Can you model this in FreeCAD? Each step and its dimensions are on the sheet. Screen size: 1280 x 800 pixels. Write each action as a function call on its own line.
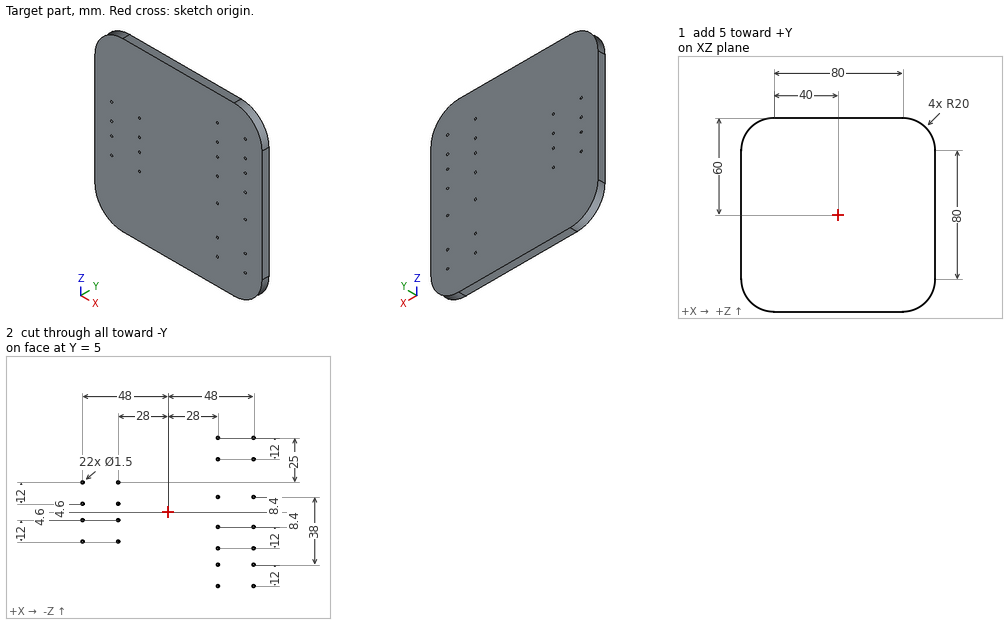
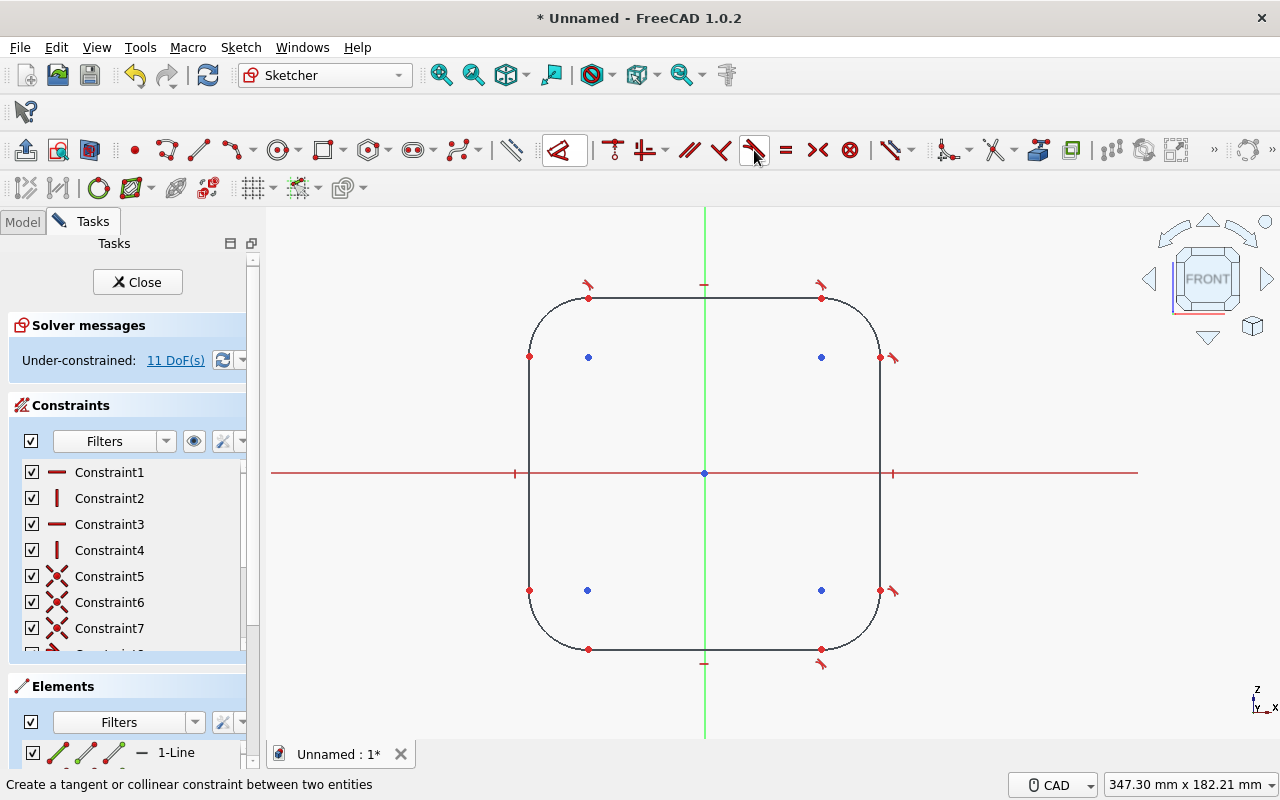
click(751, 650)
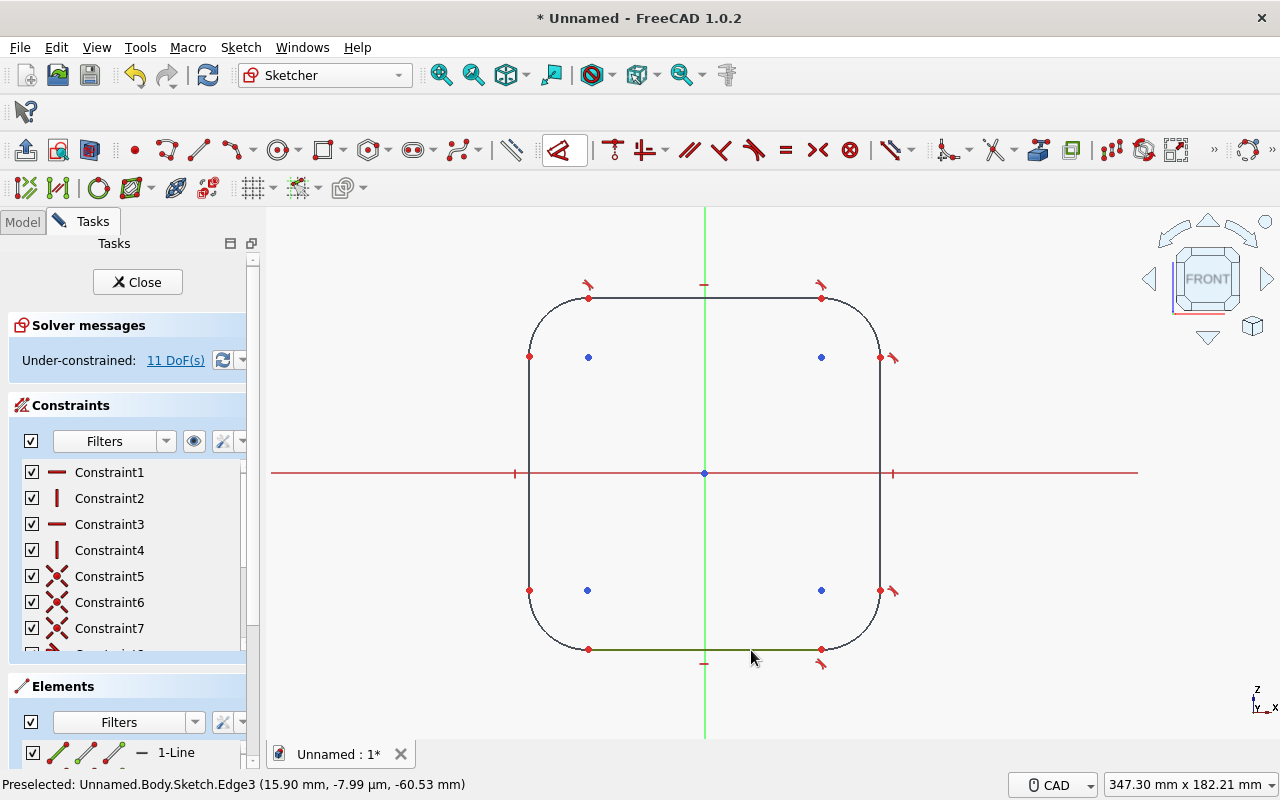
click(535, 618)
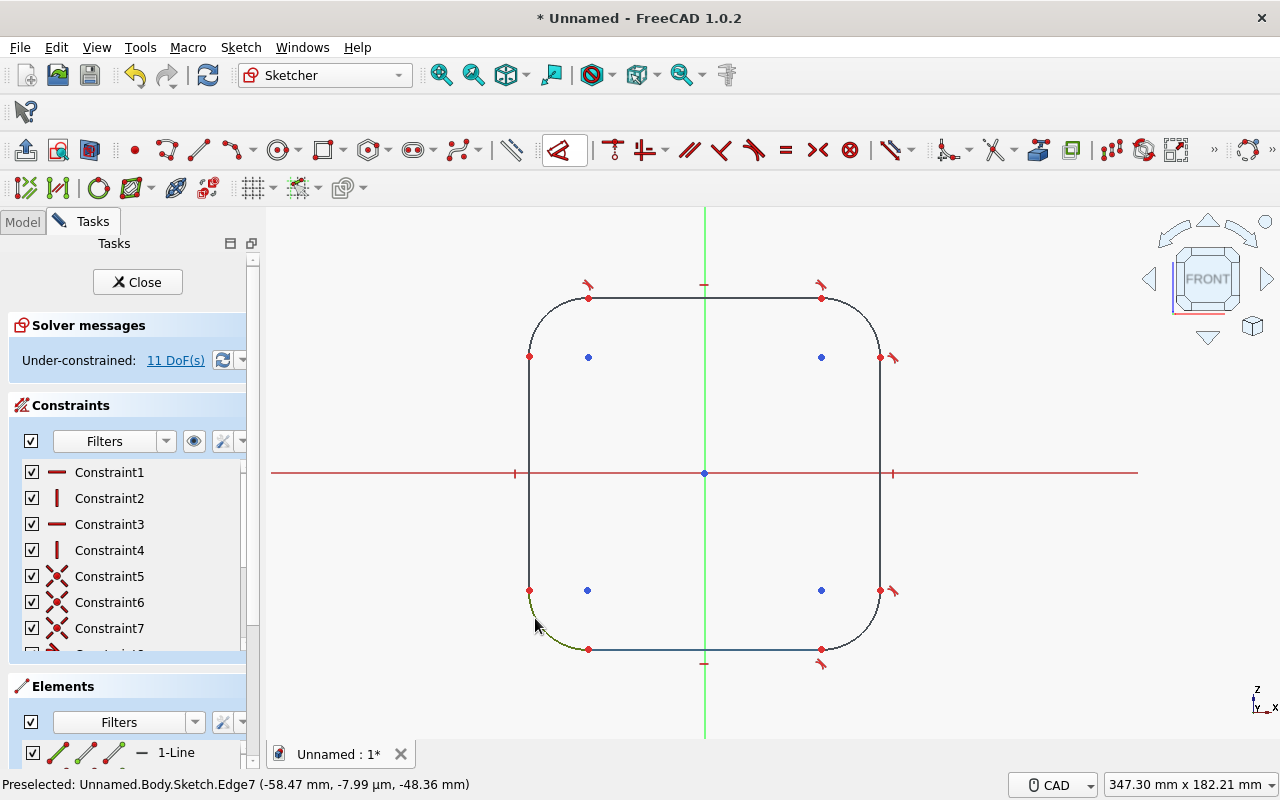
click(754, 150)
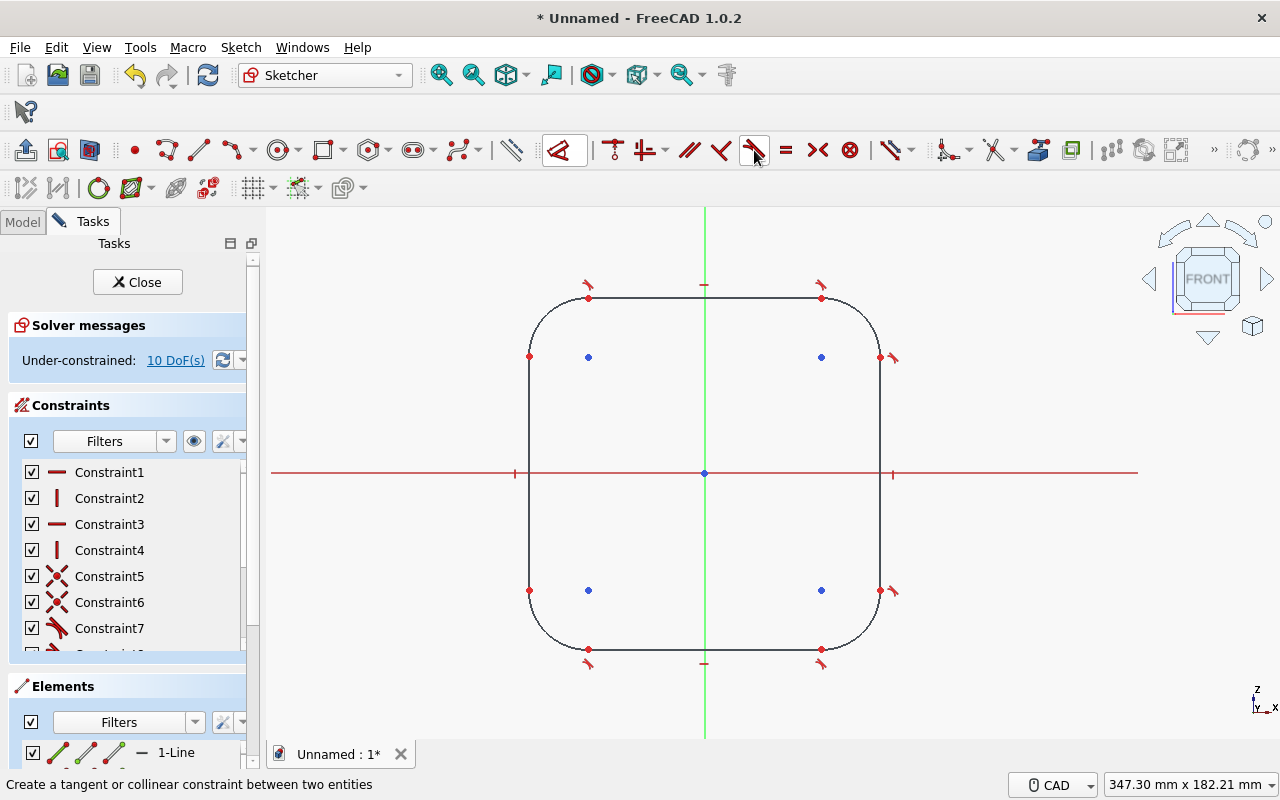
click(529, 521)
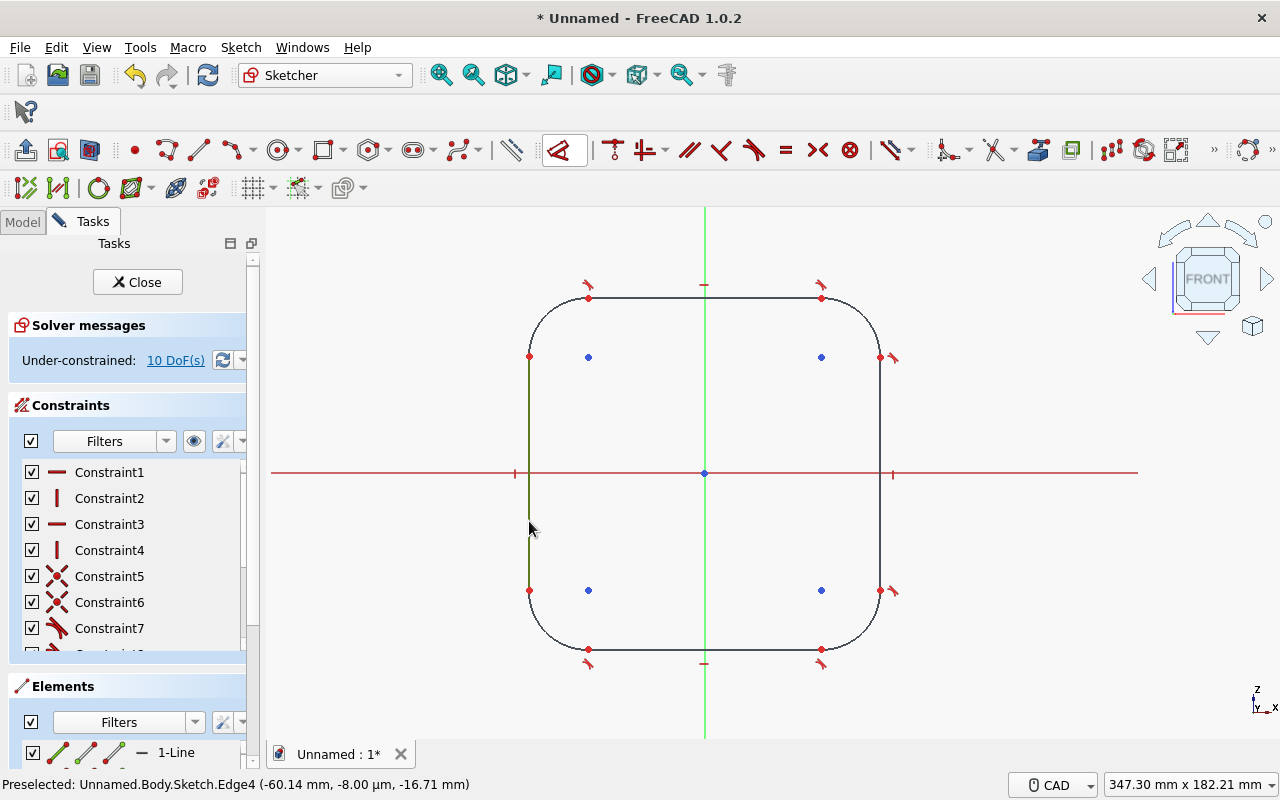
click(535, 618)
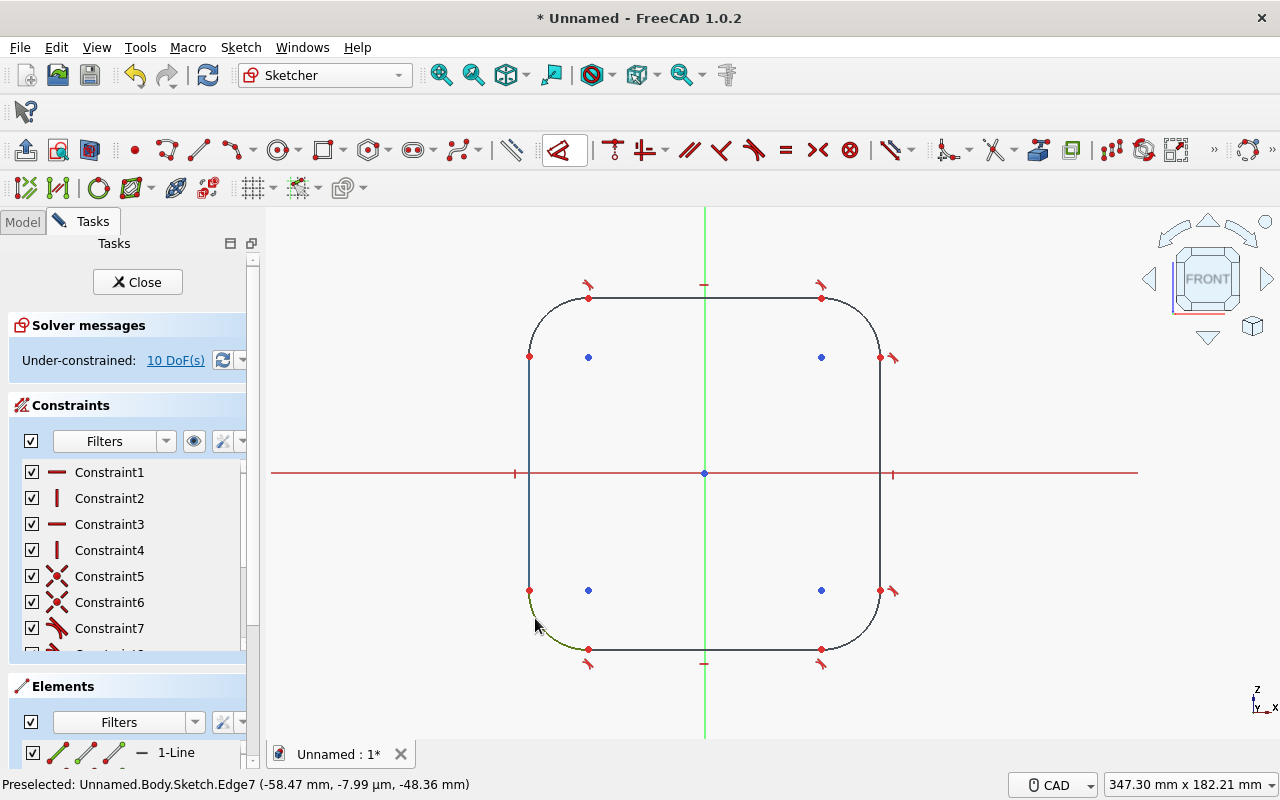
click(754, 150)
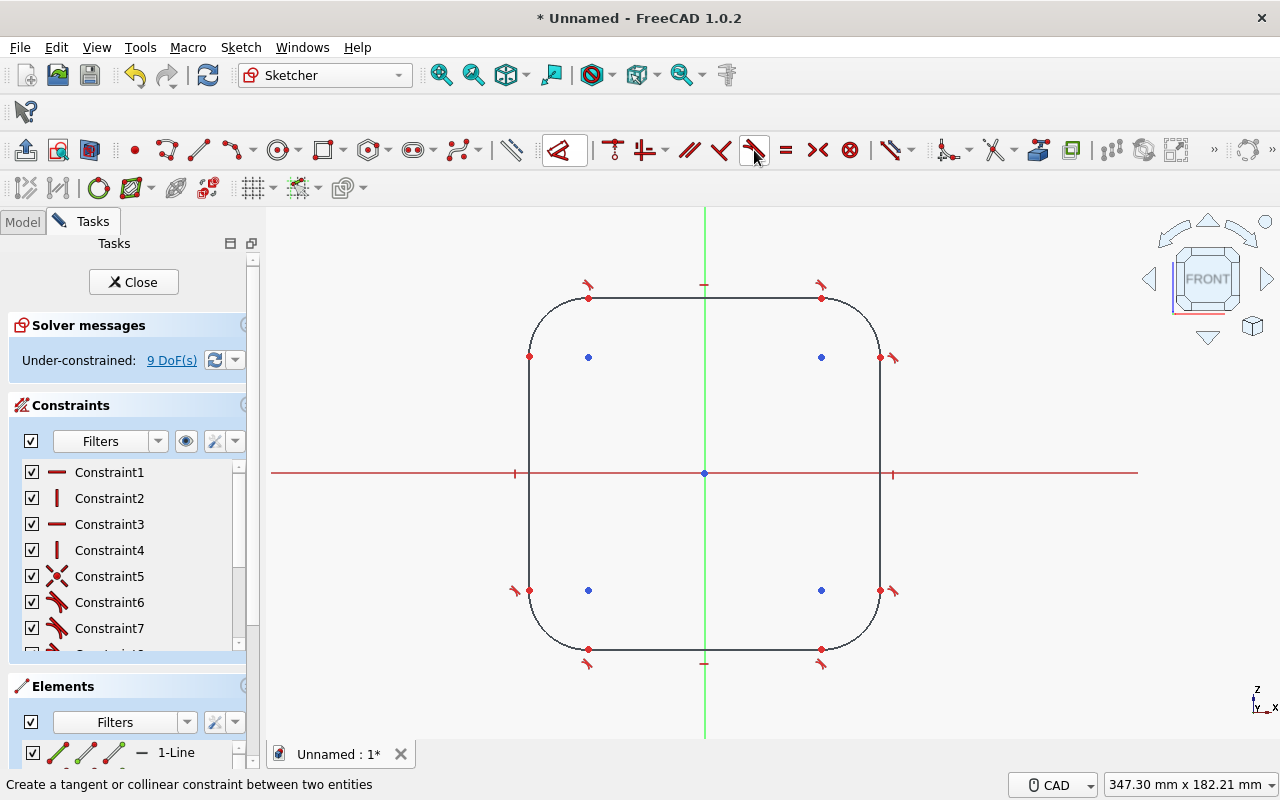
click(529, 521)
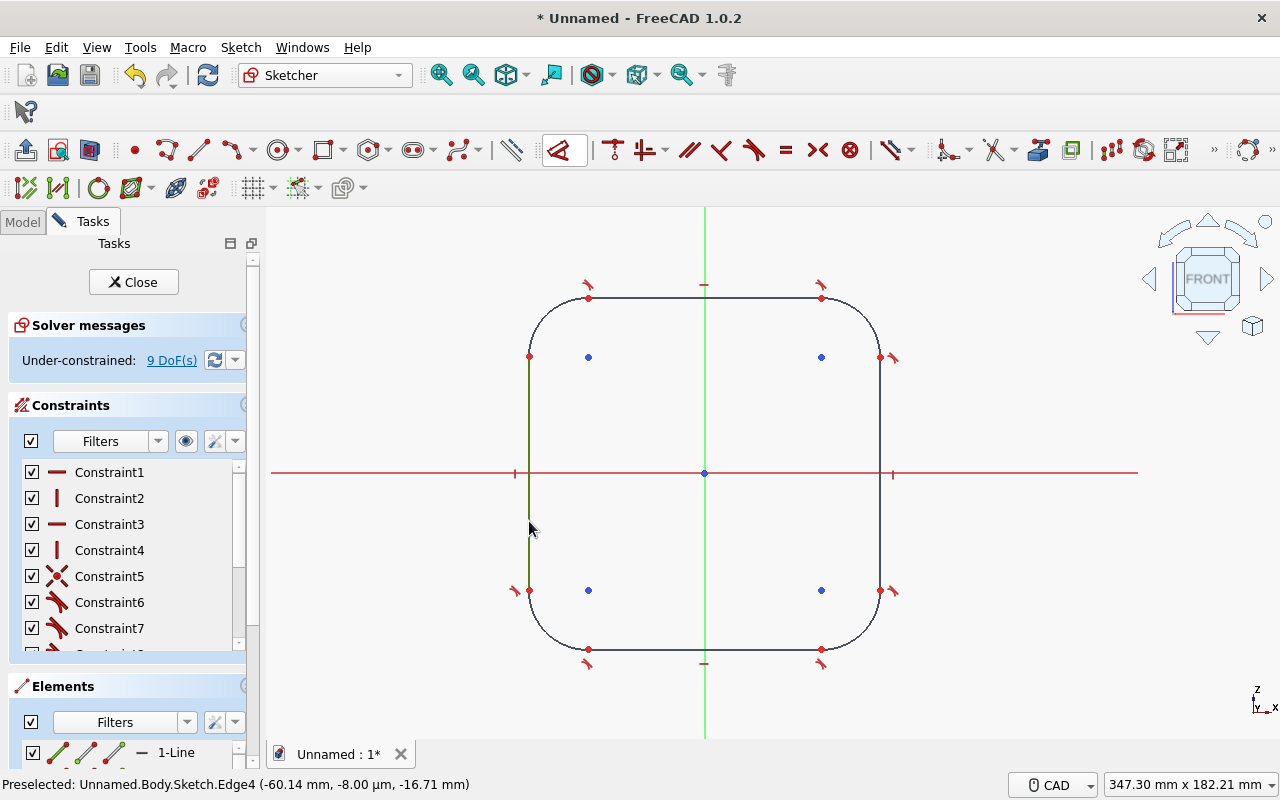
click(561, 304)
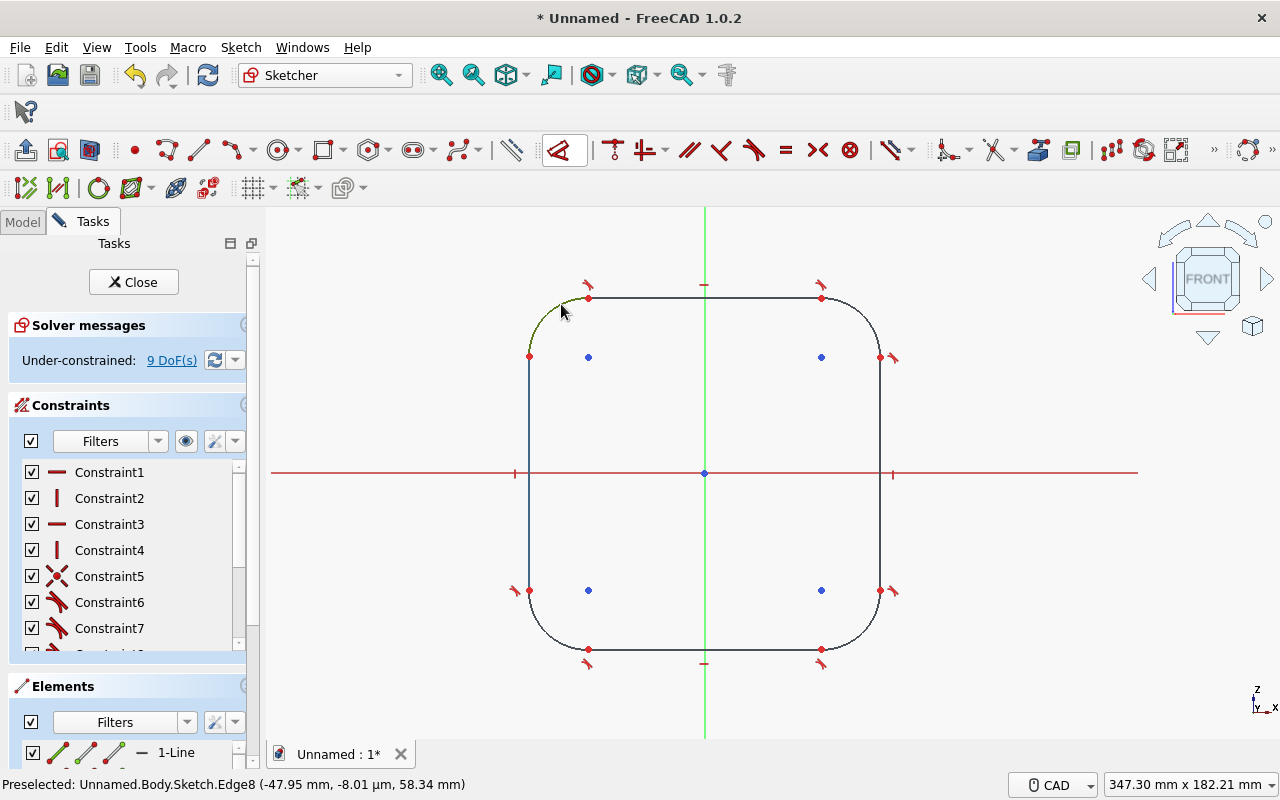
click(754, 150)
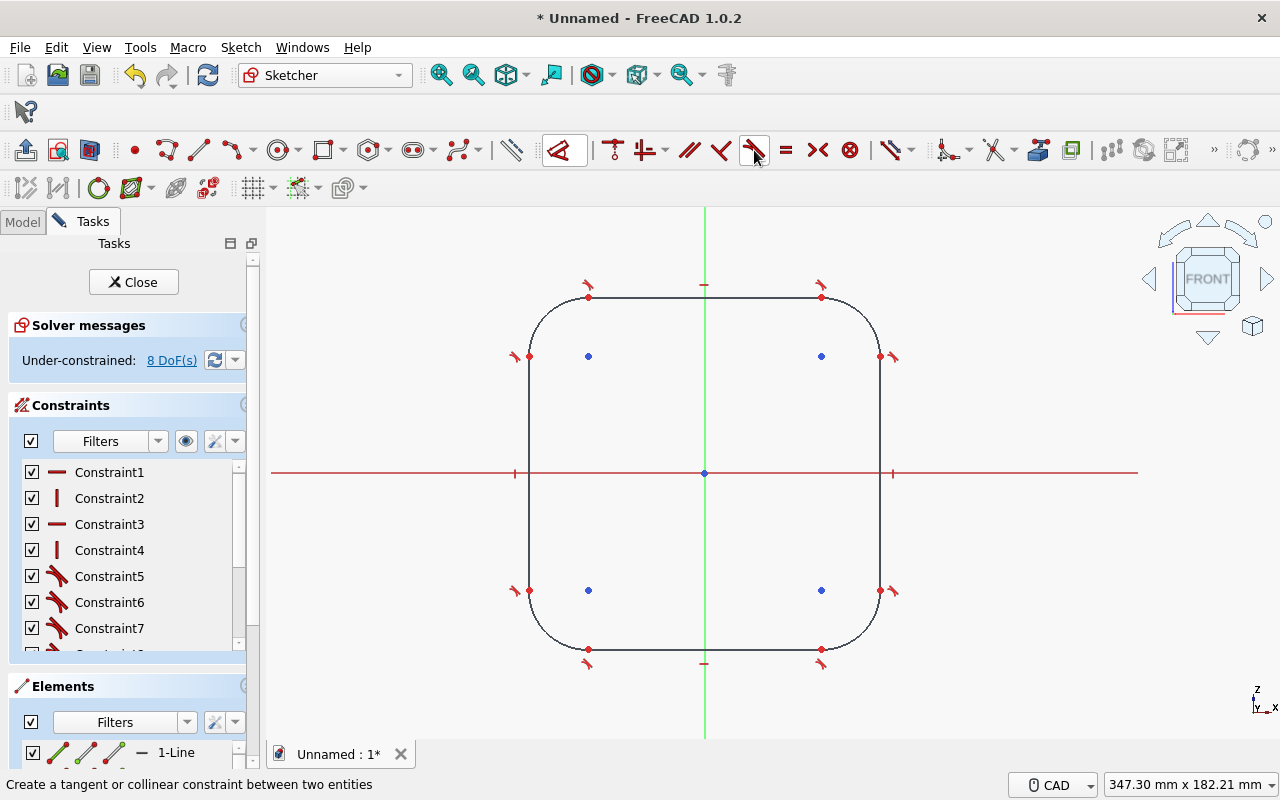
click(874, 330)